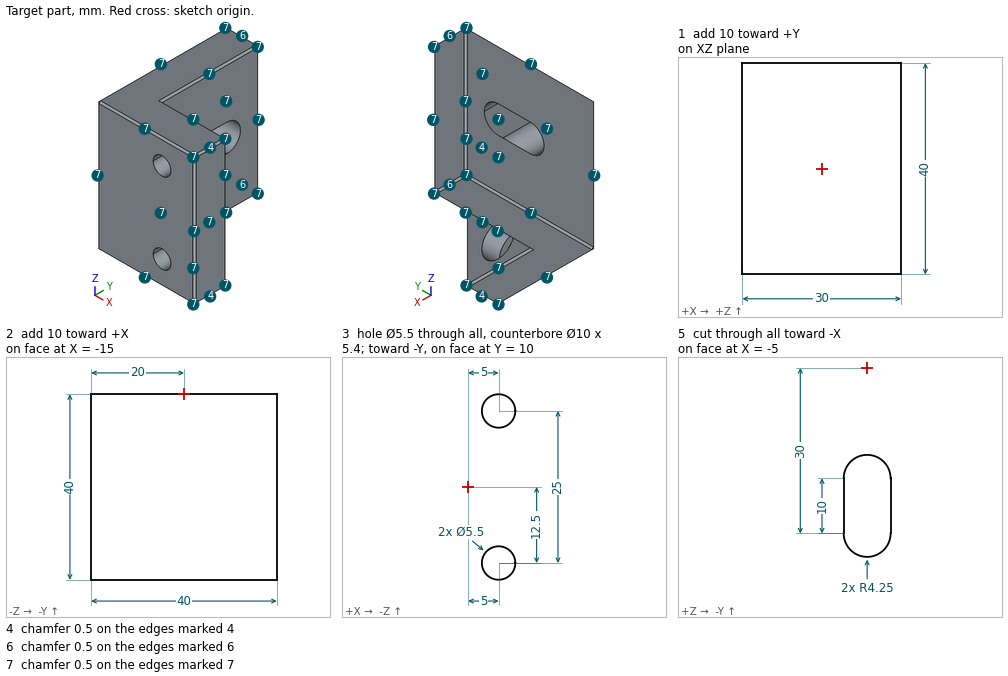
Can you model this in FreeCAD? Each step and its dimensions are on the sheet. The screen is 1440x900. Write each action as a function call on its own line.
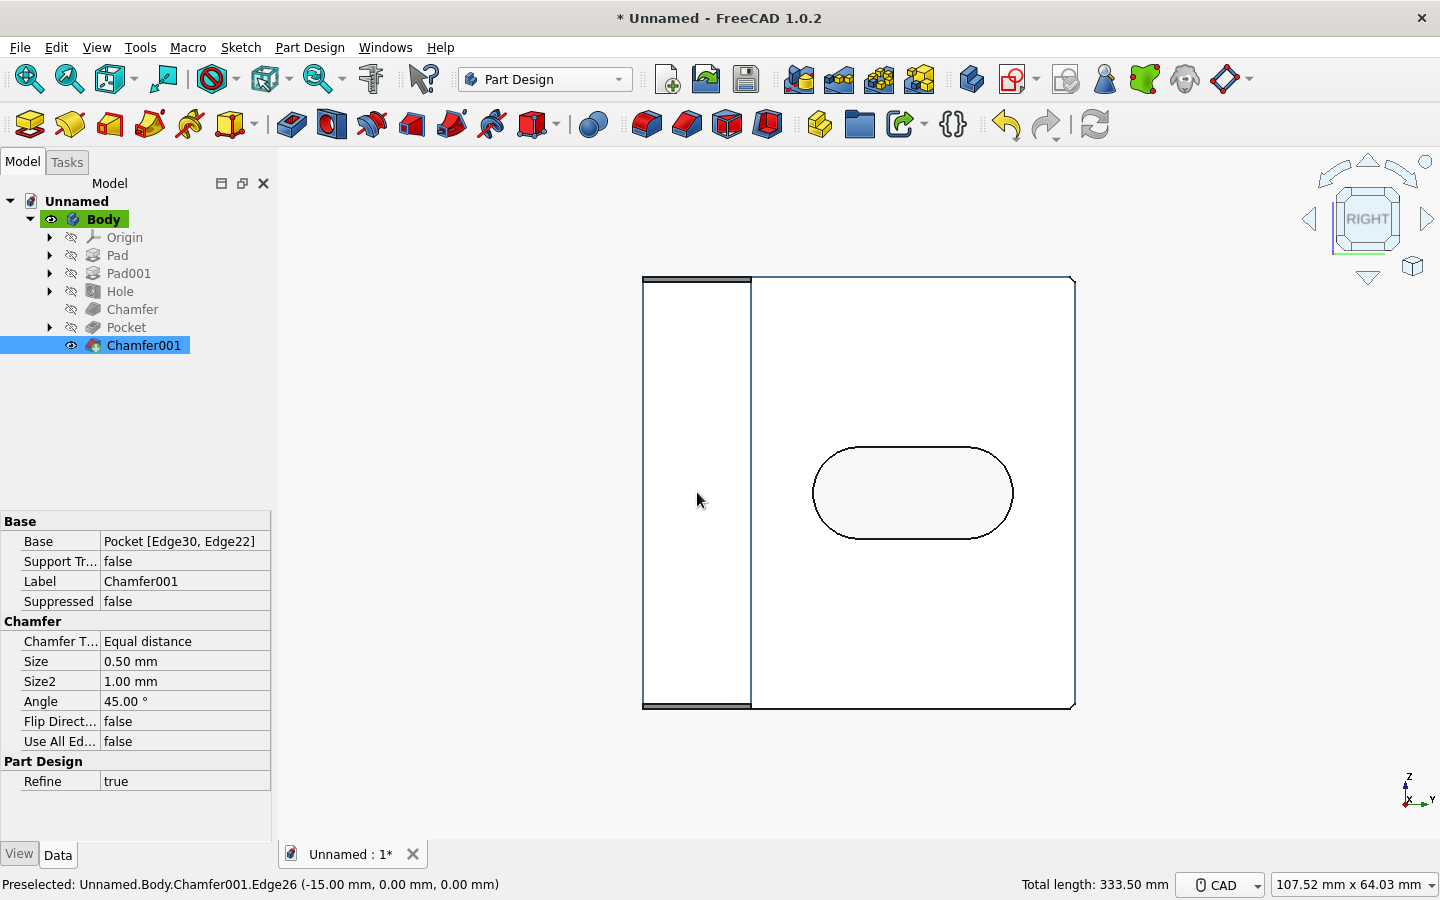
click(910, 708, ctrl)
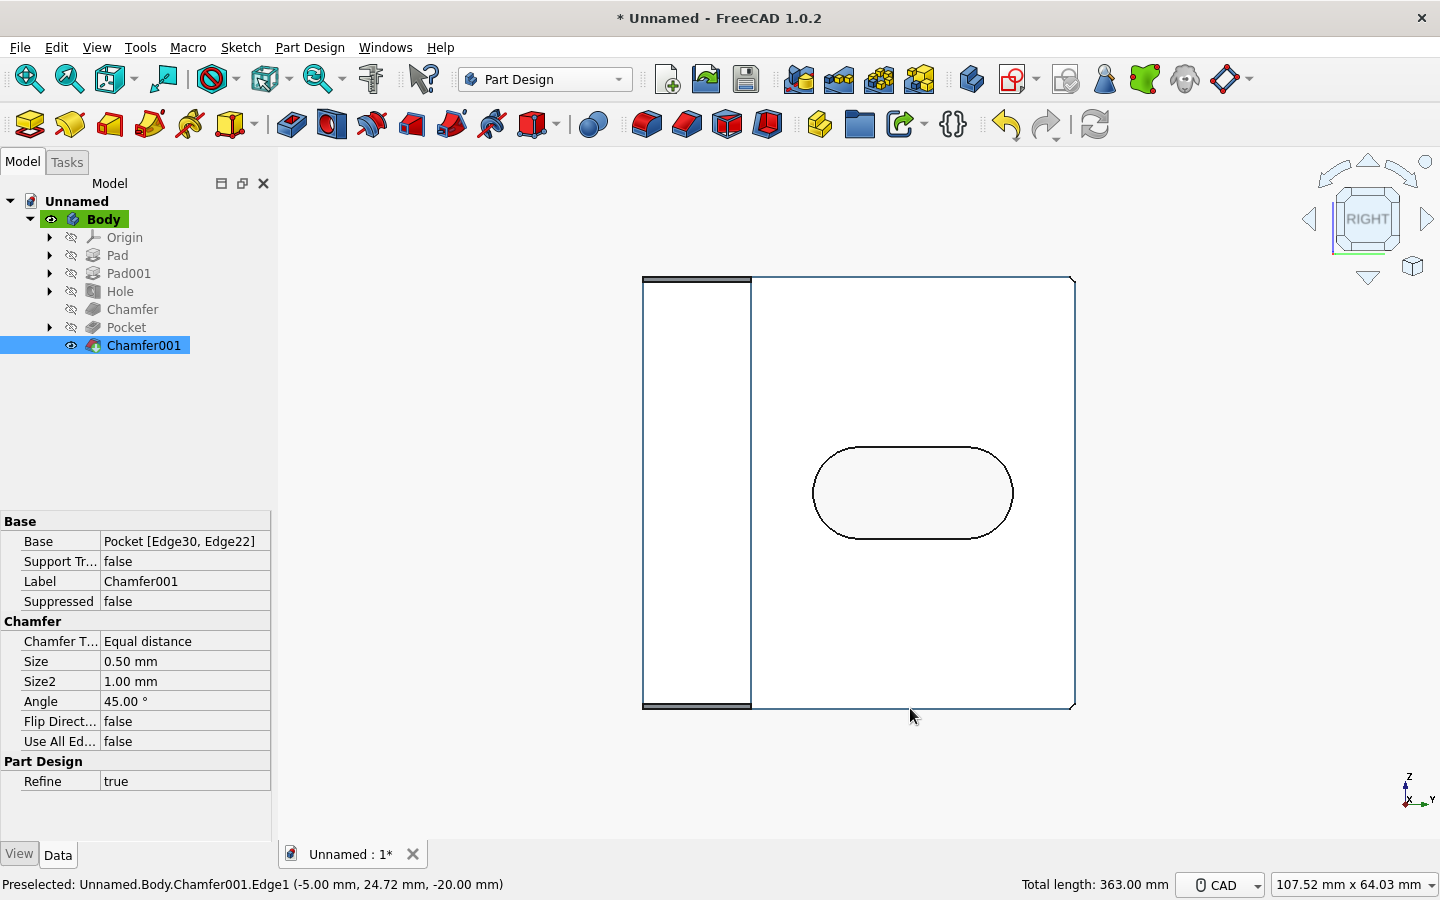
key(5)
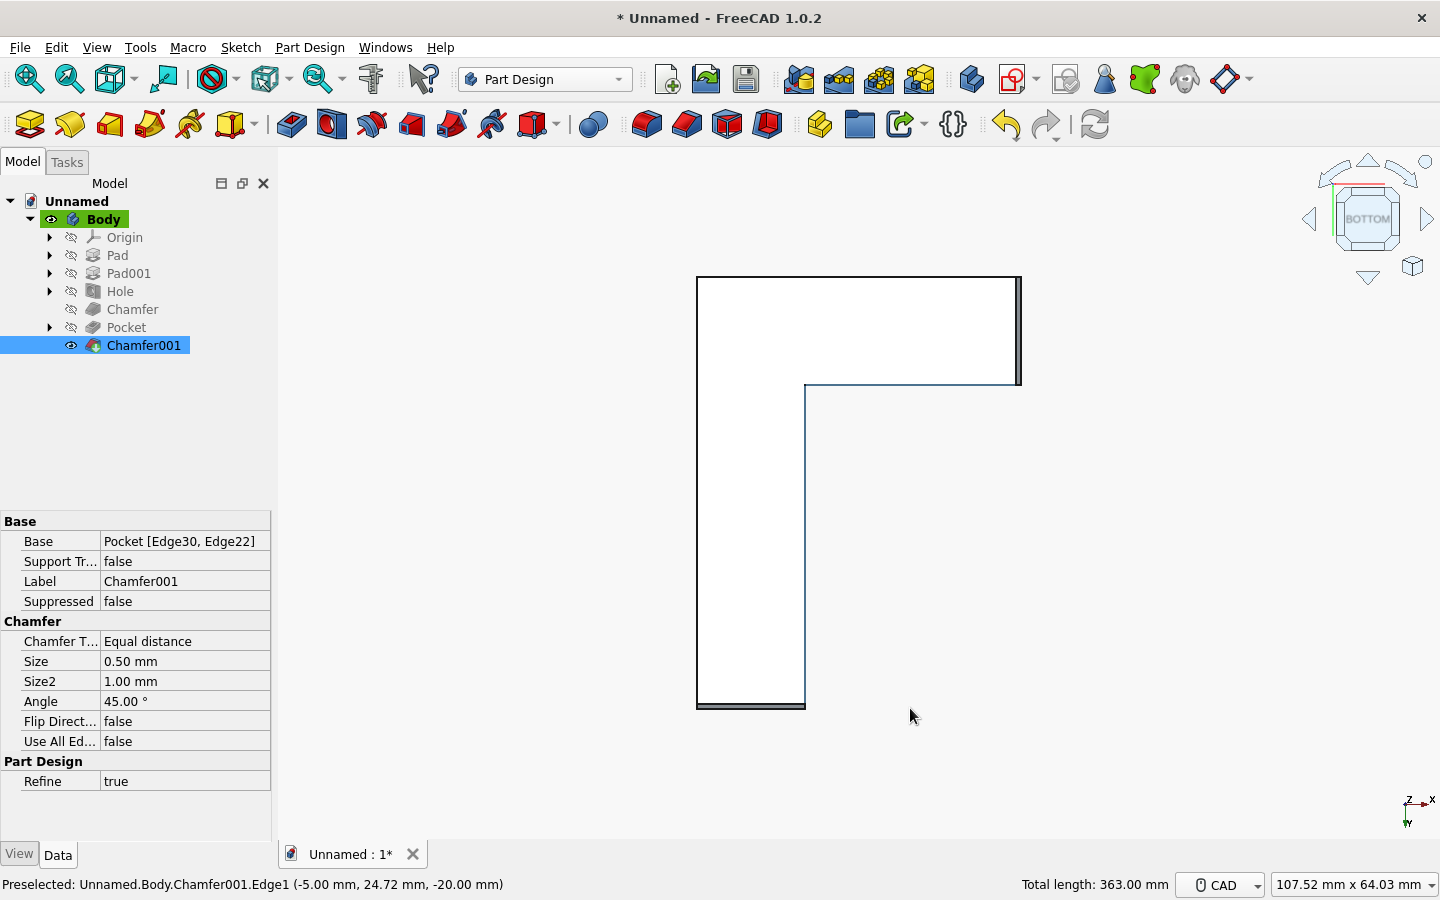
click(856, 276, ctrl)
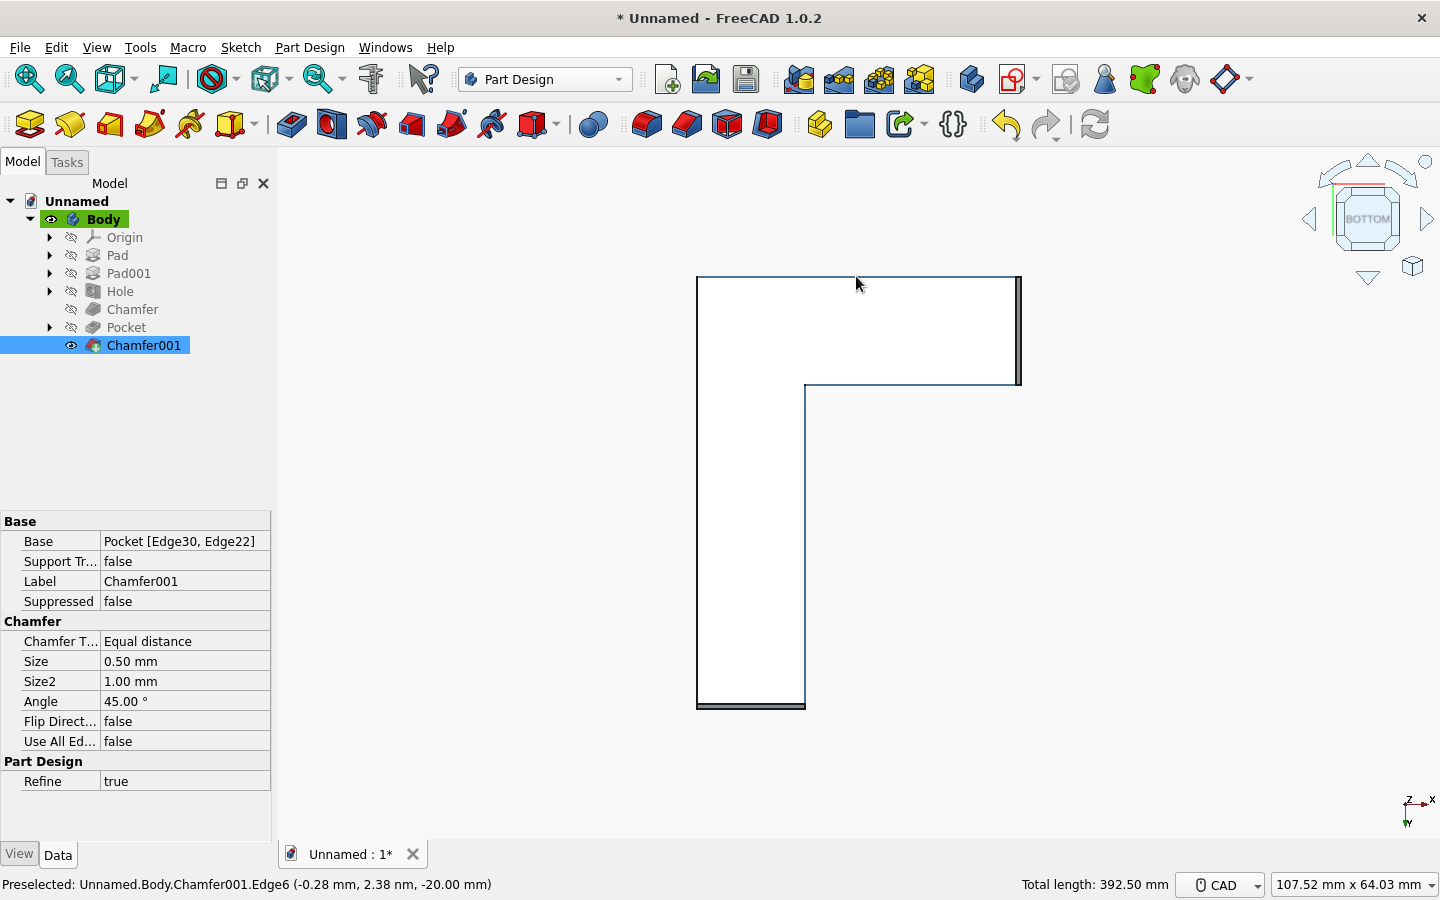
click(697, 489, ctrl)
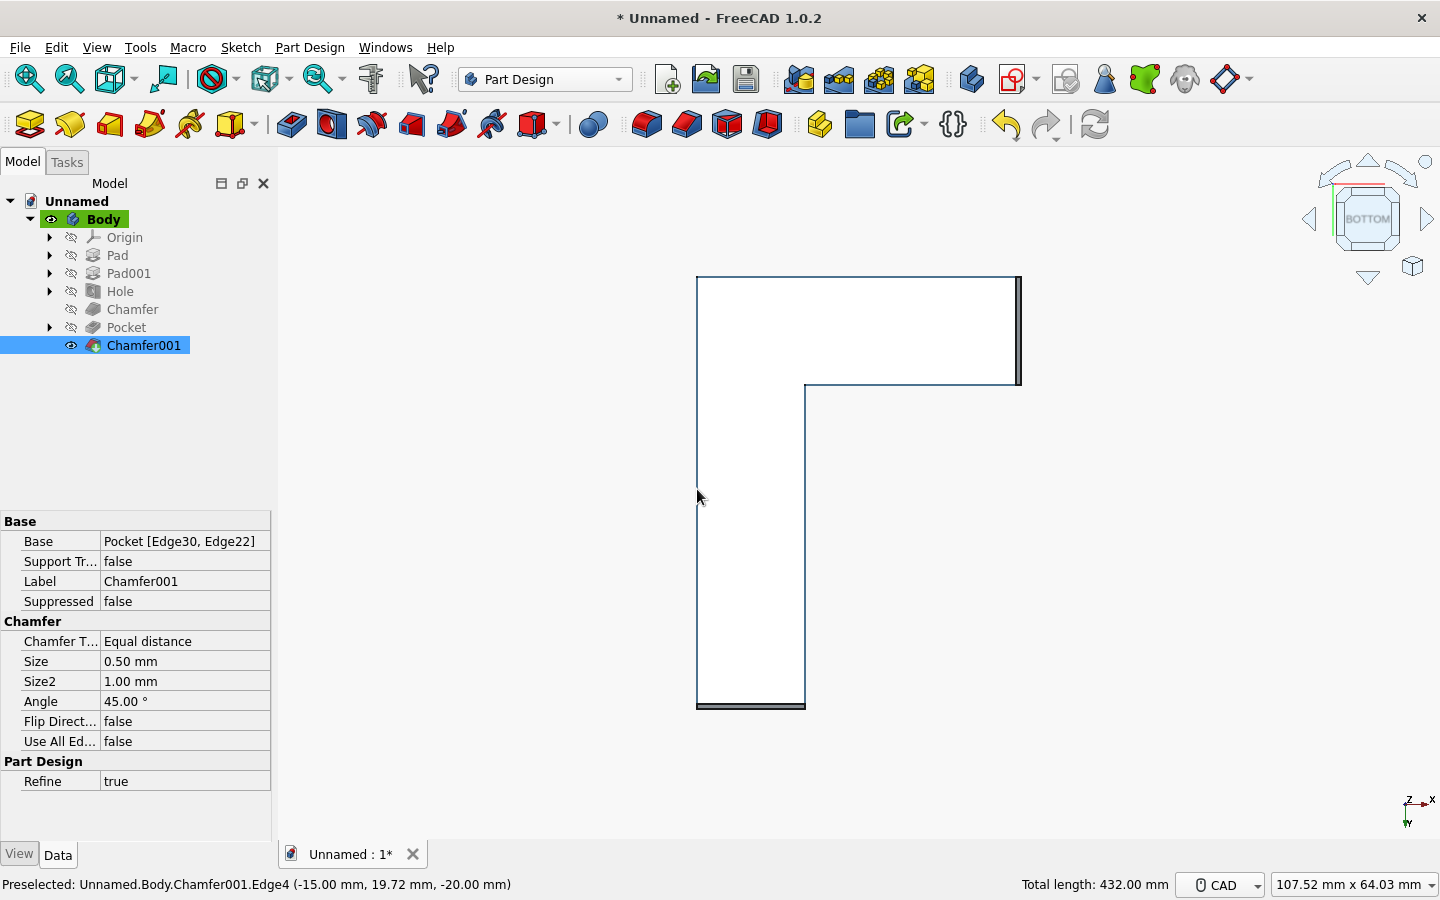
scroll(1018, 276, up, 9)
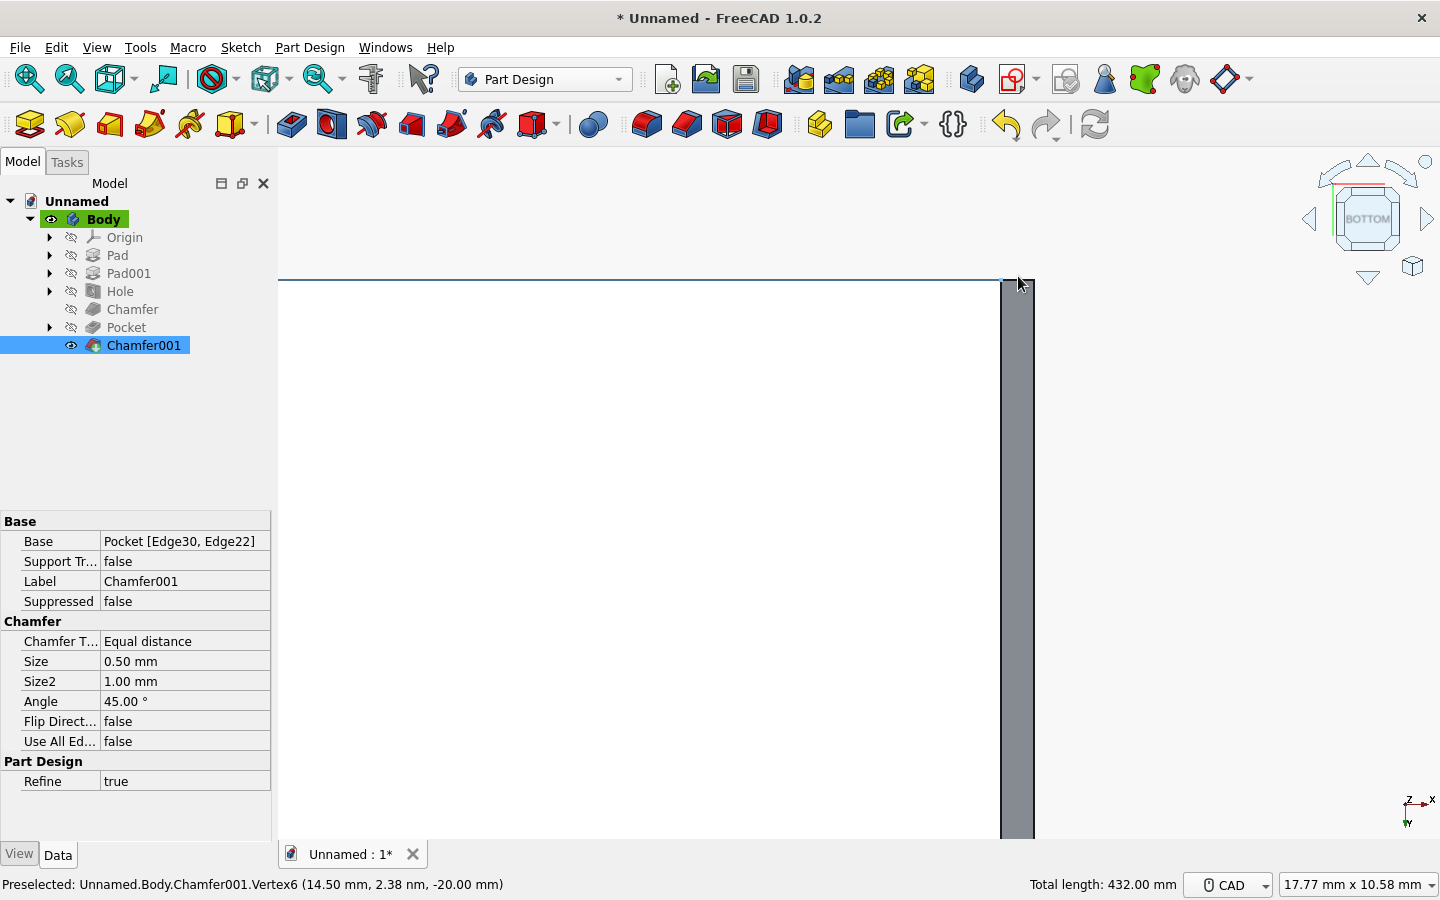
click(1017, 279, ctrl)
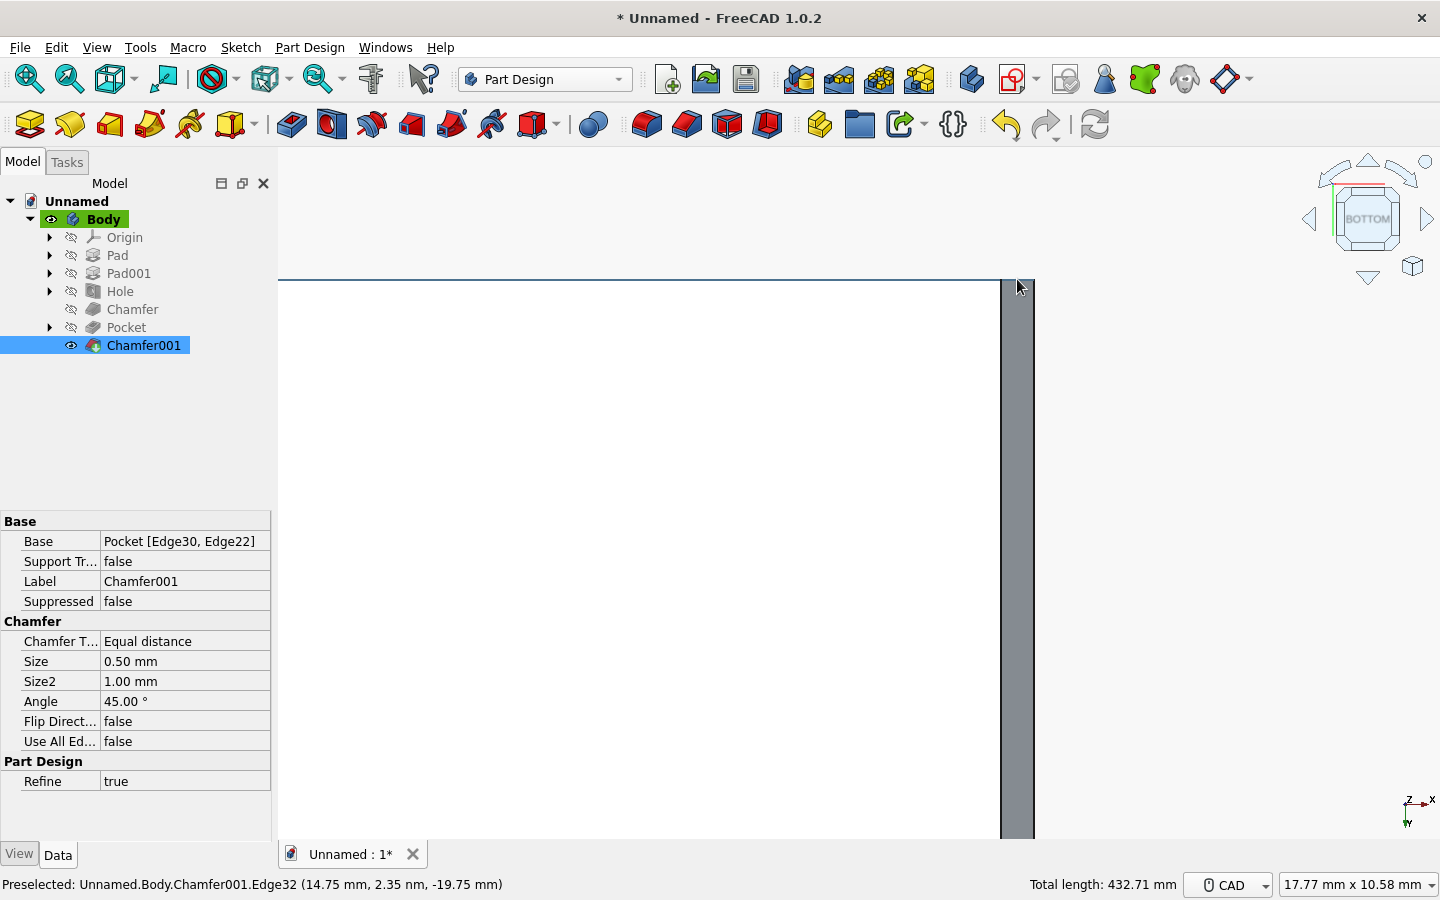
click(30, 80)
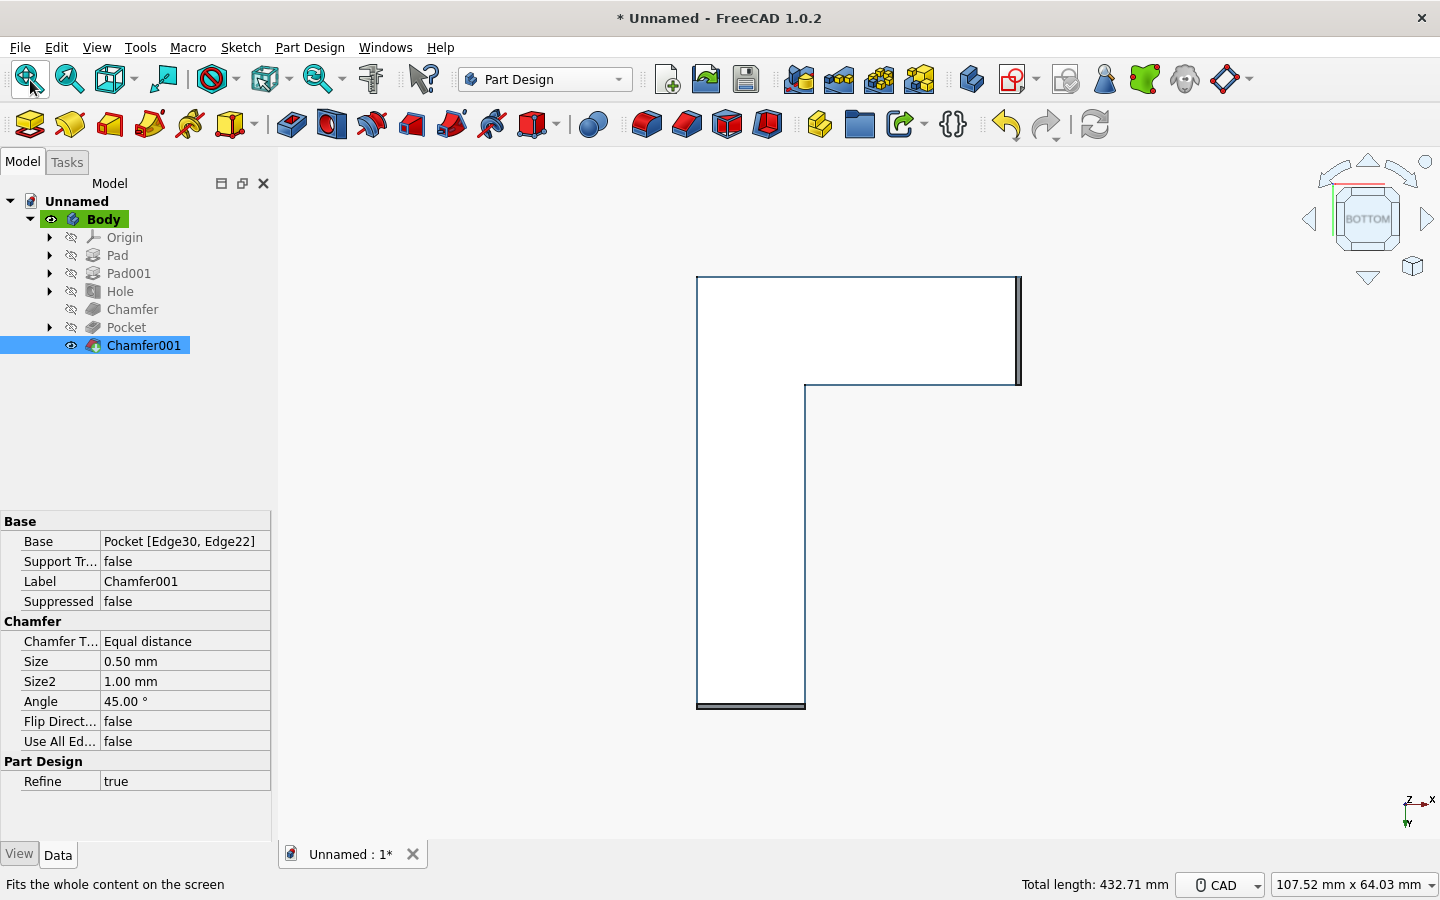
key(4)